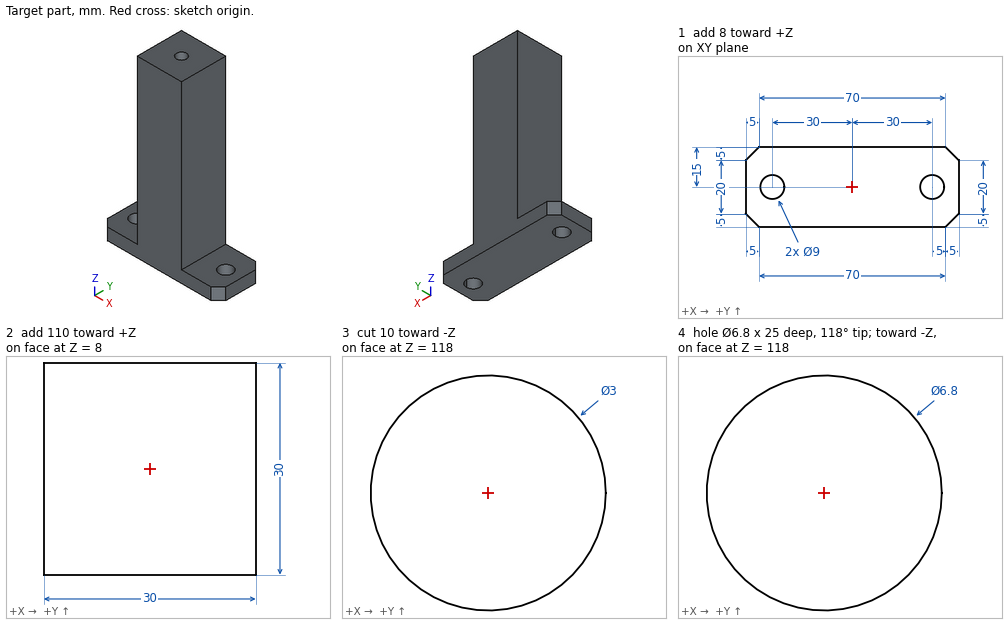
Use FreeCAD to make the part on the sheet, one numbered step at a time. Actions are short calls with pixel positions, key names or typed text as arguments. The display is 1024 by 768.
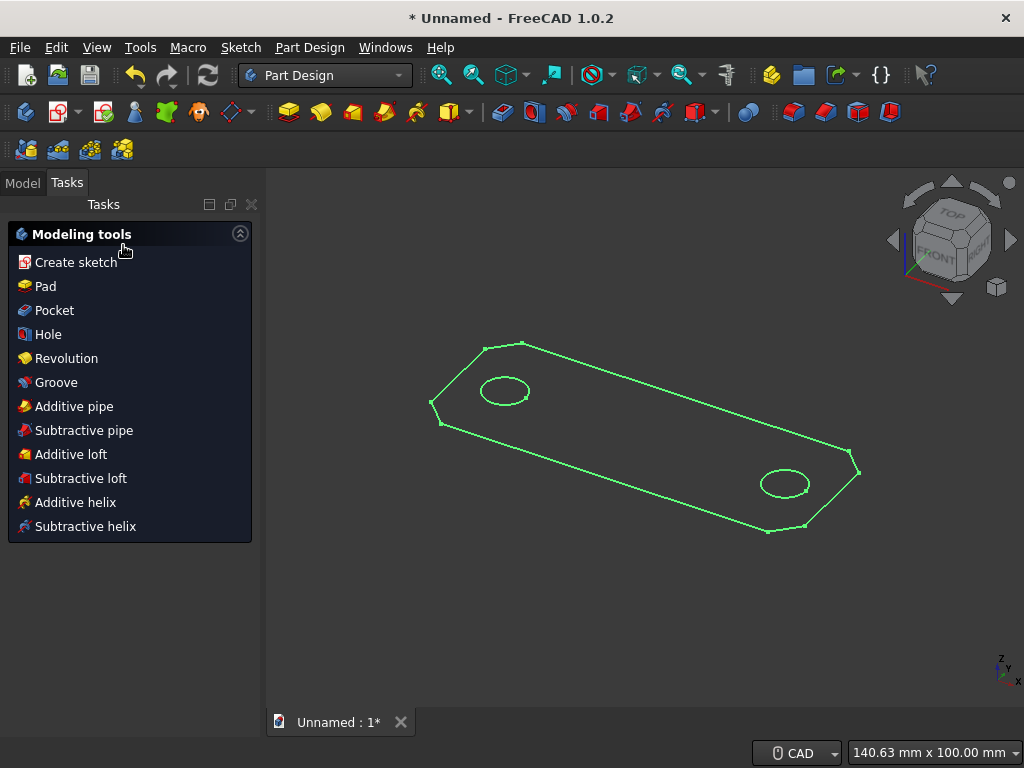
click(290, 112)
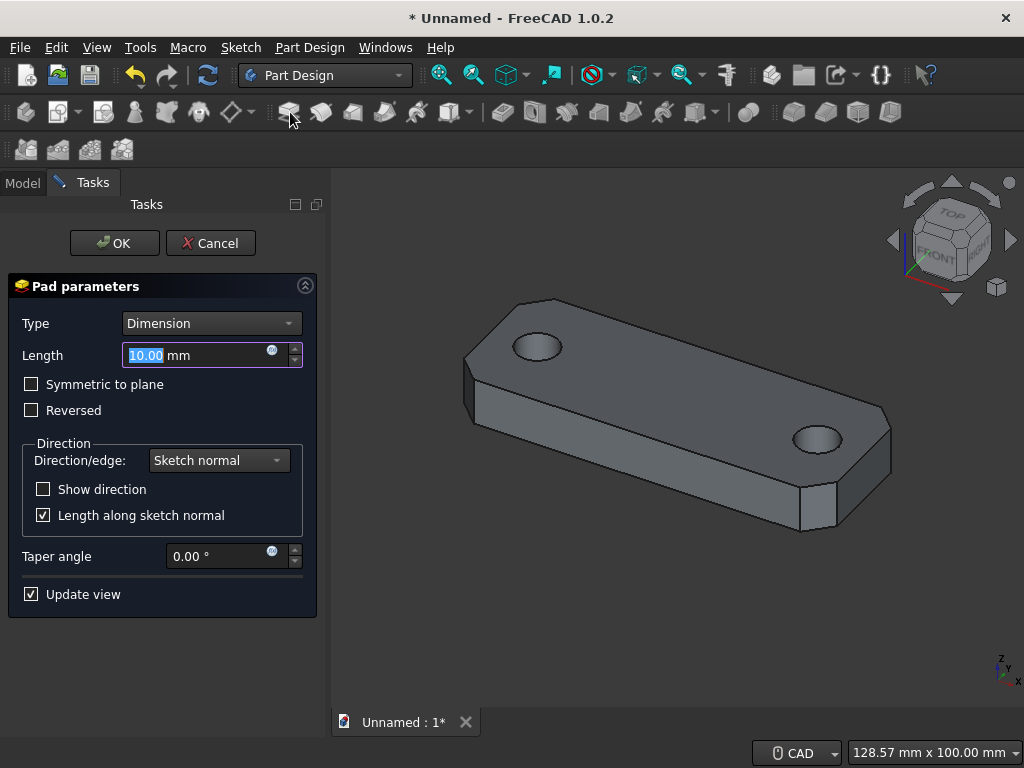
text(8)
key(Tab)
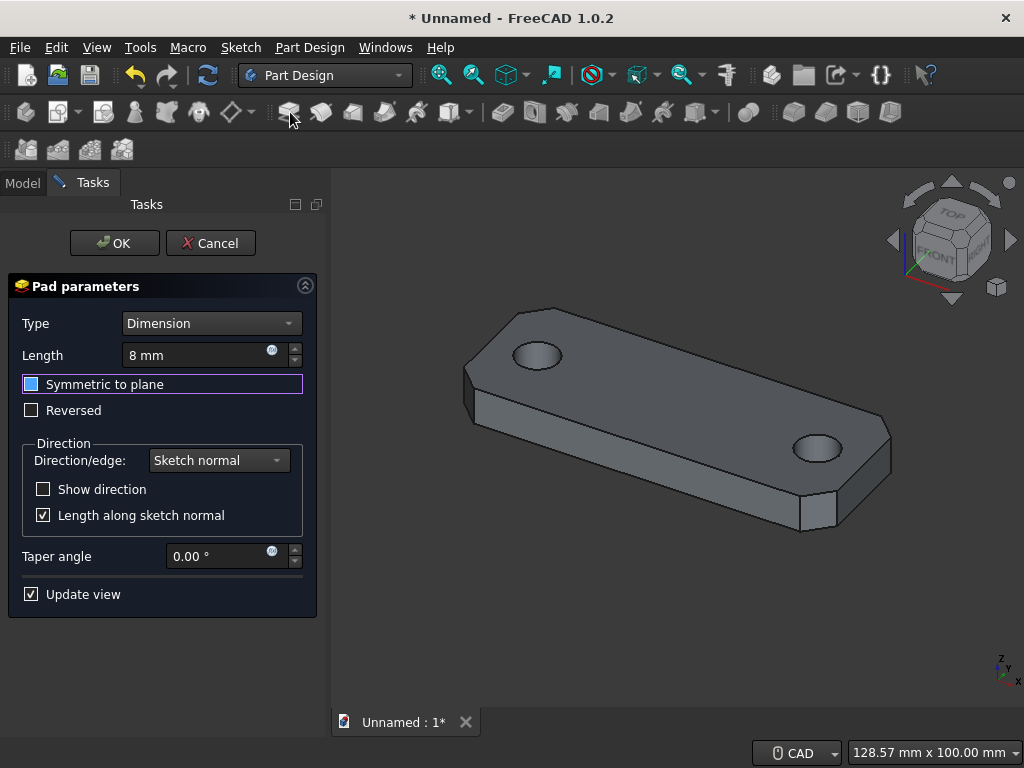
click(115, 243)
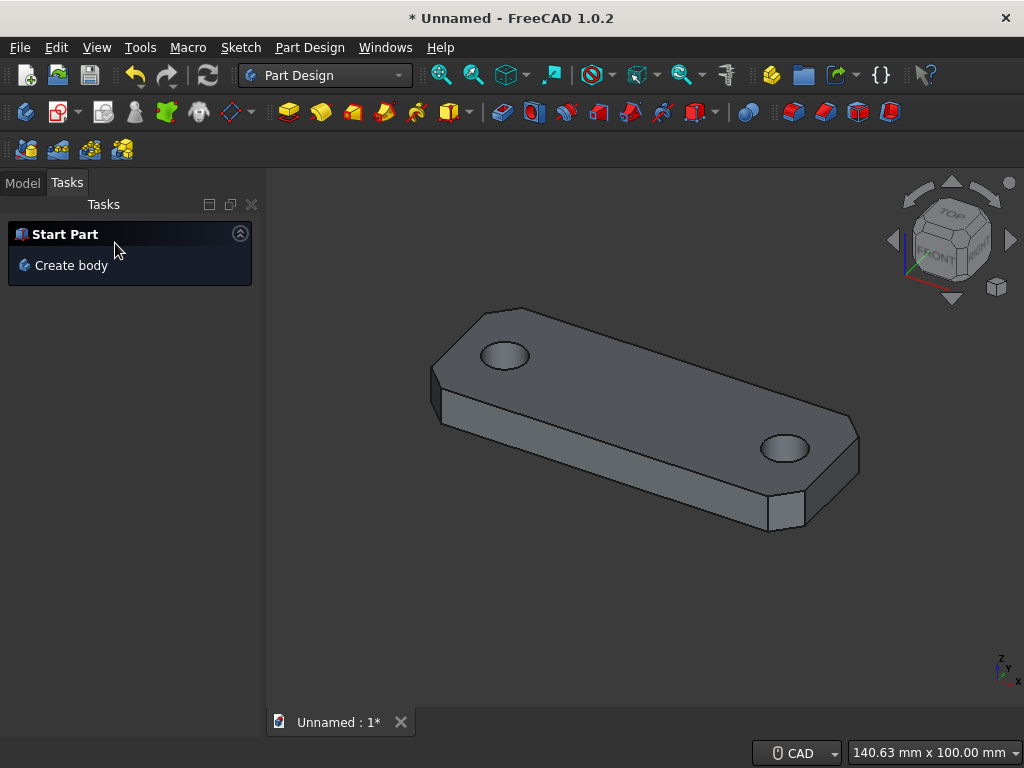
click(645, 401)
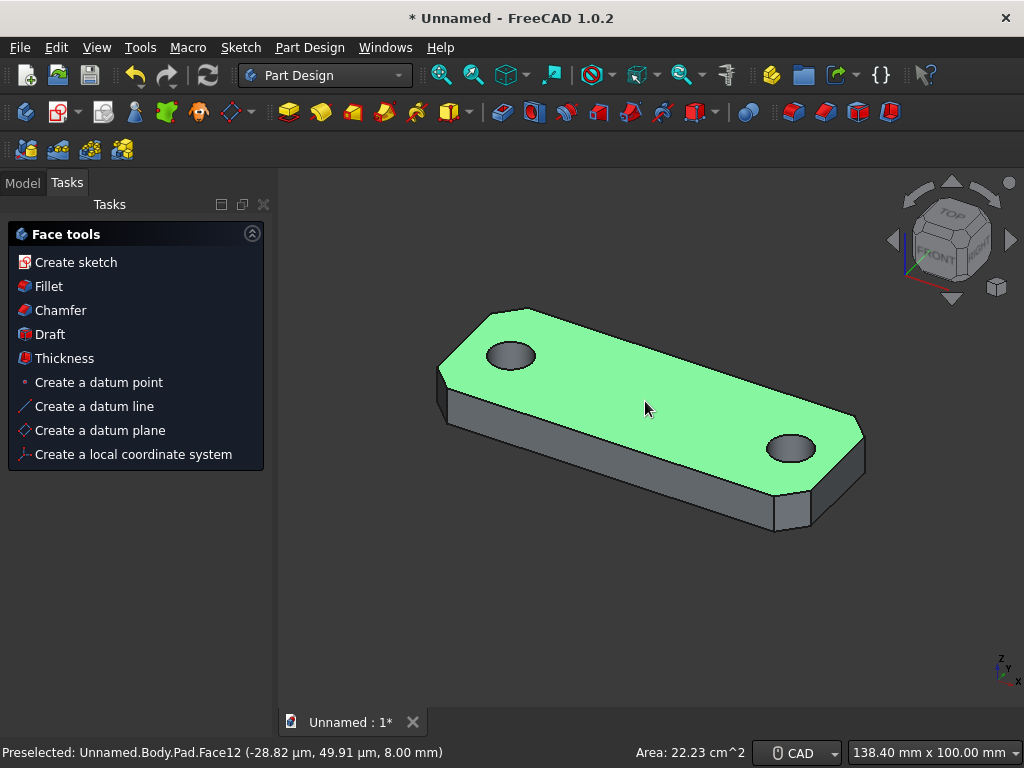
click(58, 112)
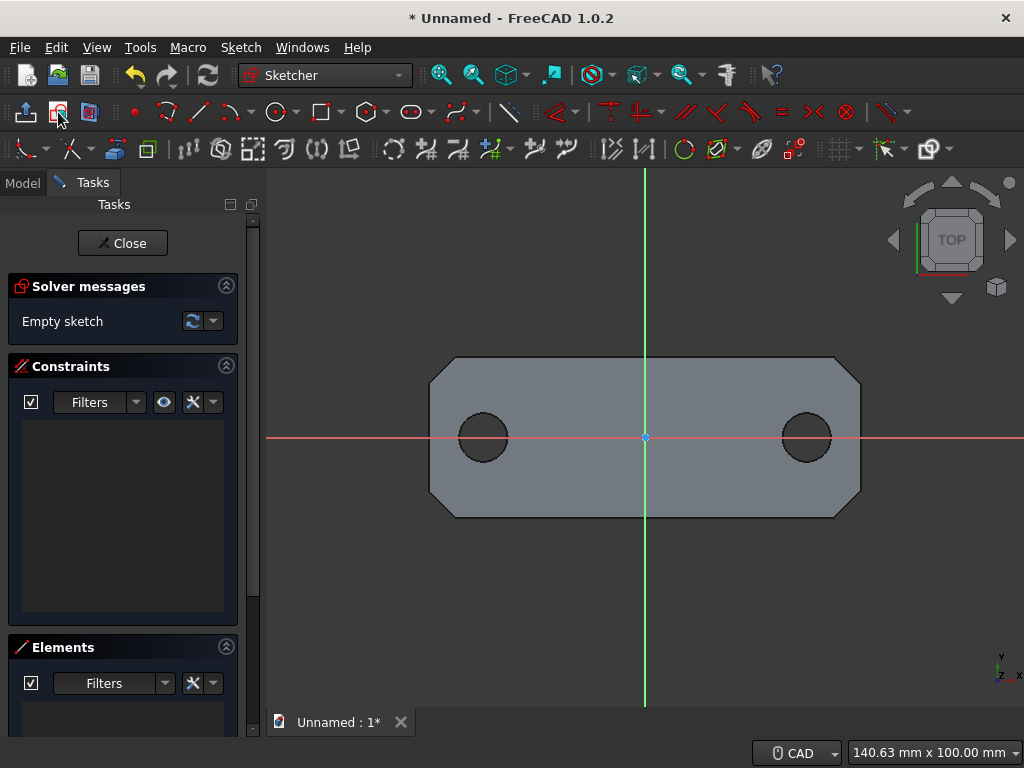
scroll(701, 438, up, 4)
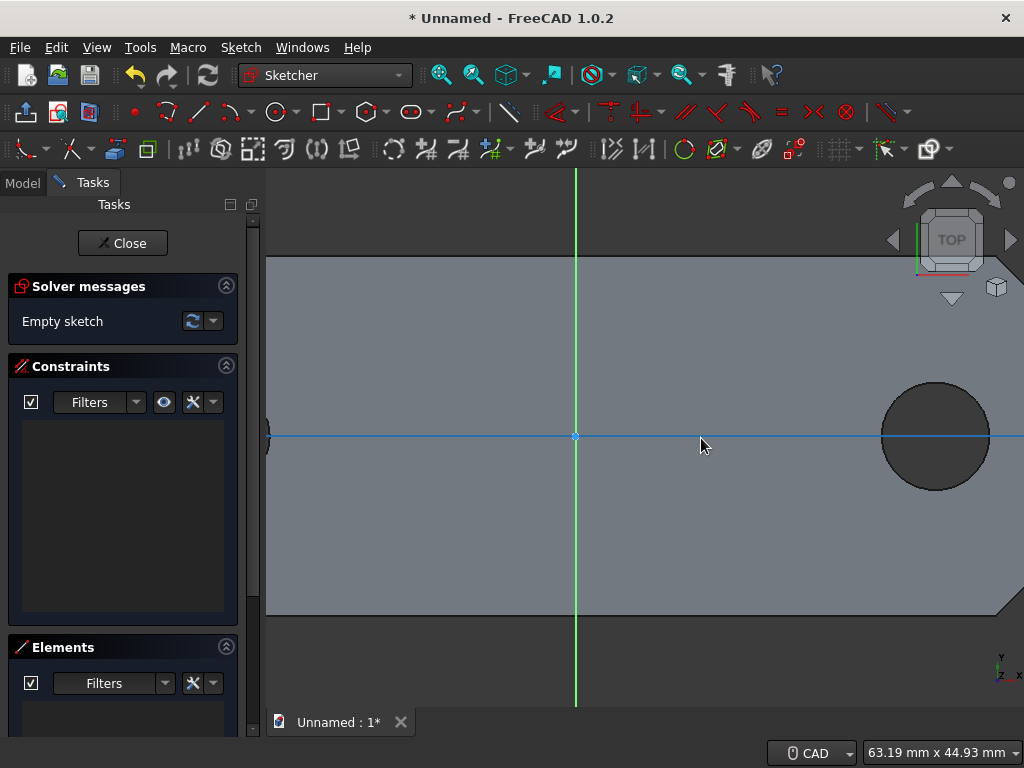
click(344, 112)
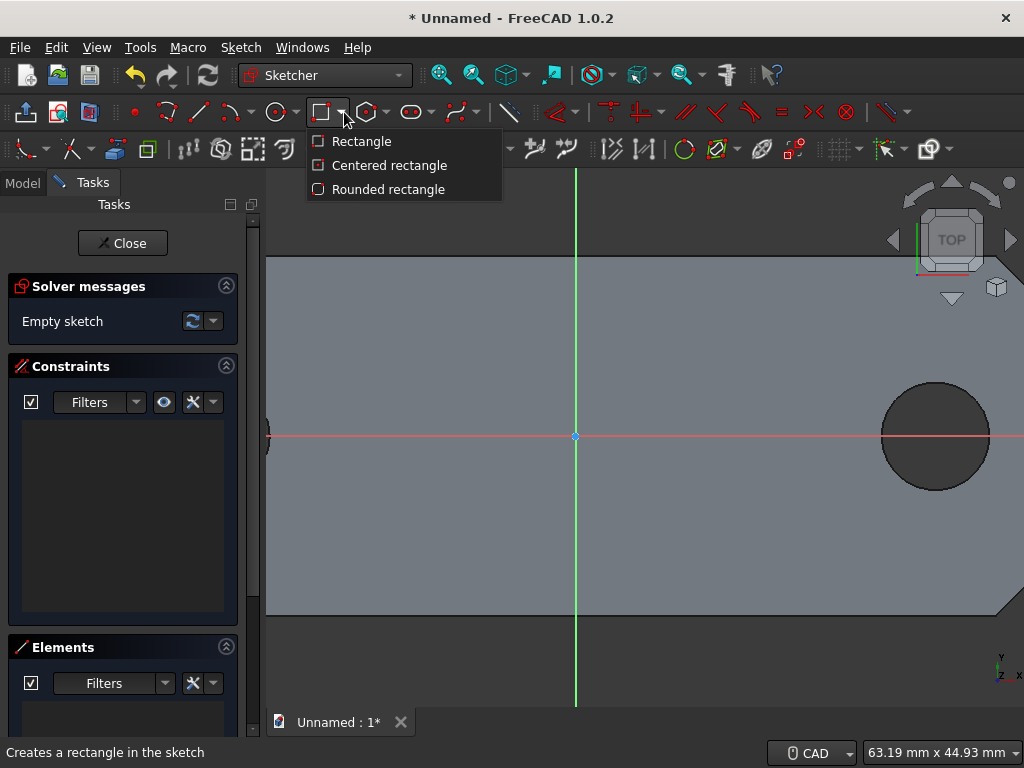
click(404, 165)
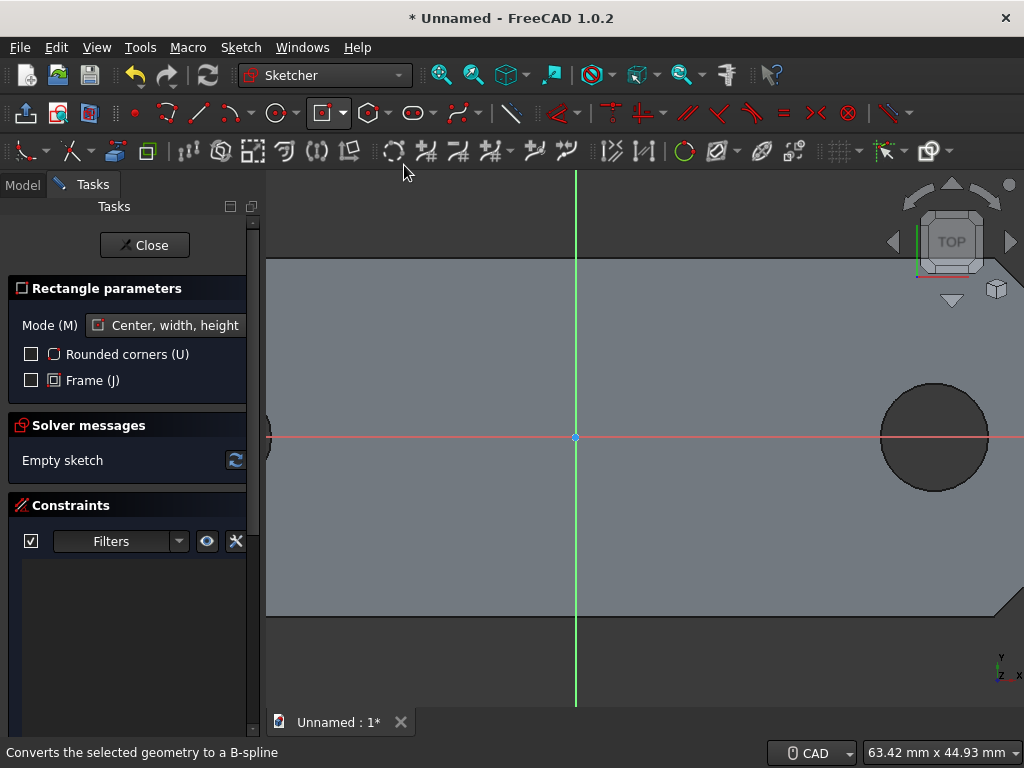
click(576, 437)
click(755, 258)
key(Escape)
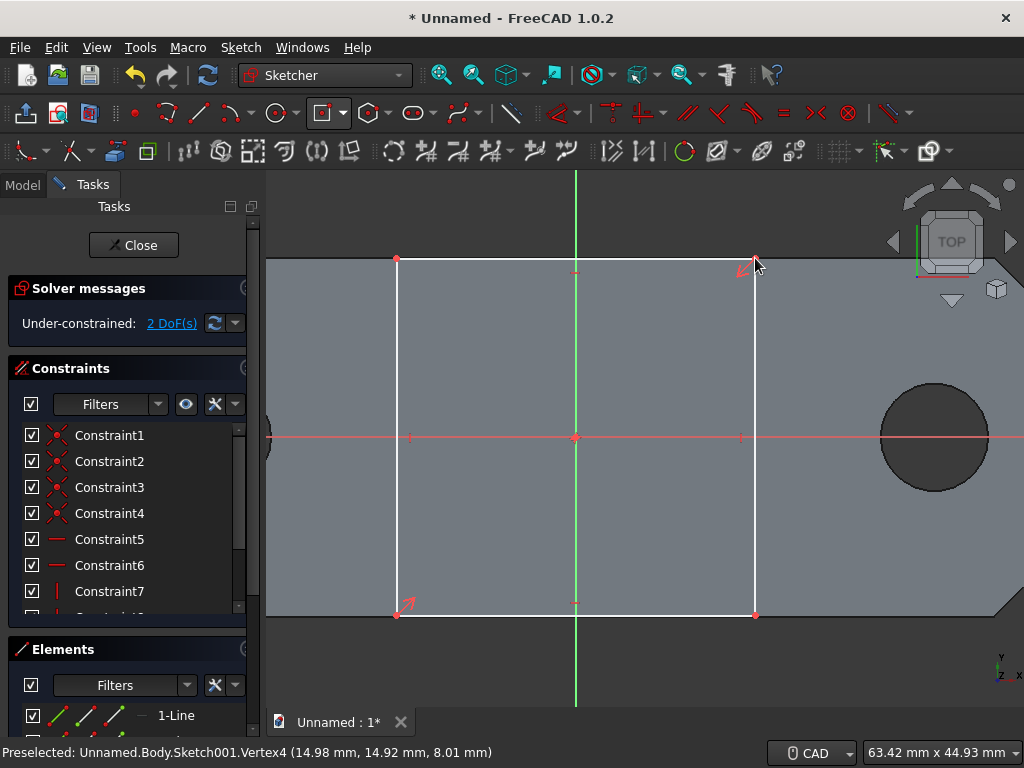
click(558, 114)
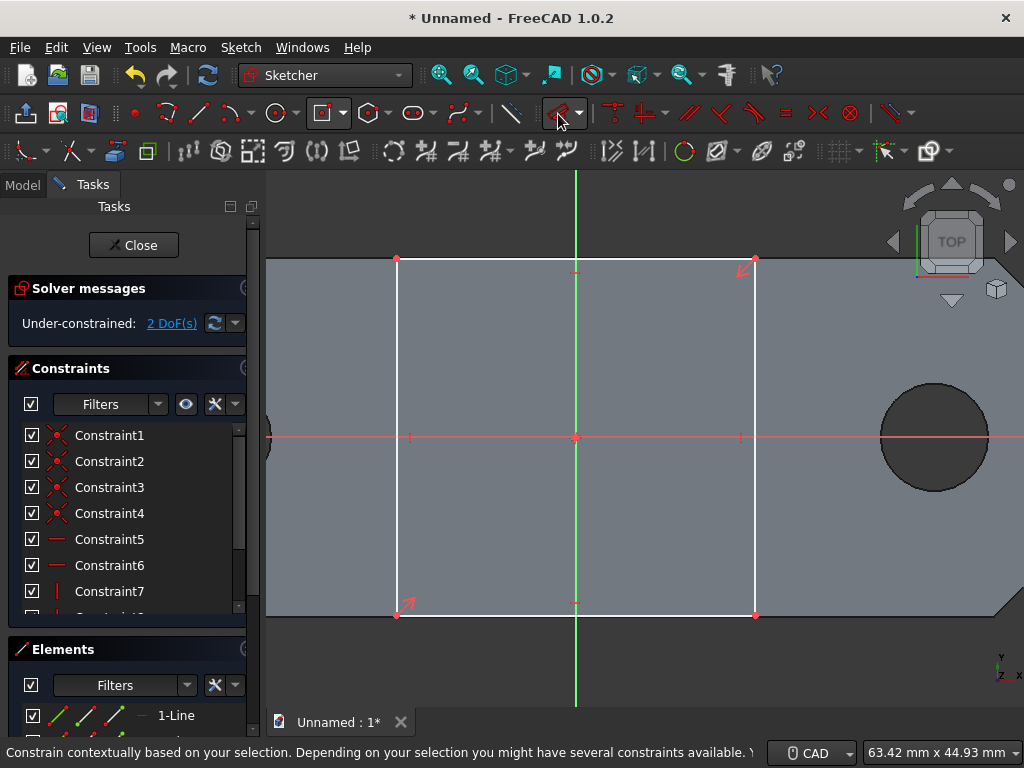
click(504, 616)
click(494, 650)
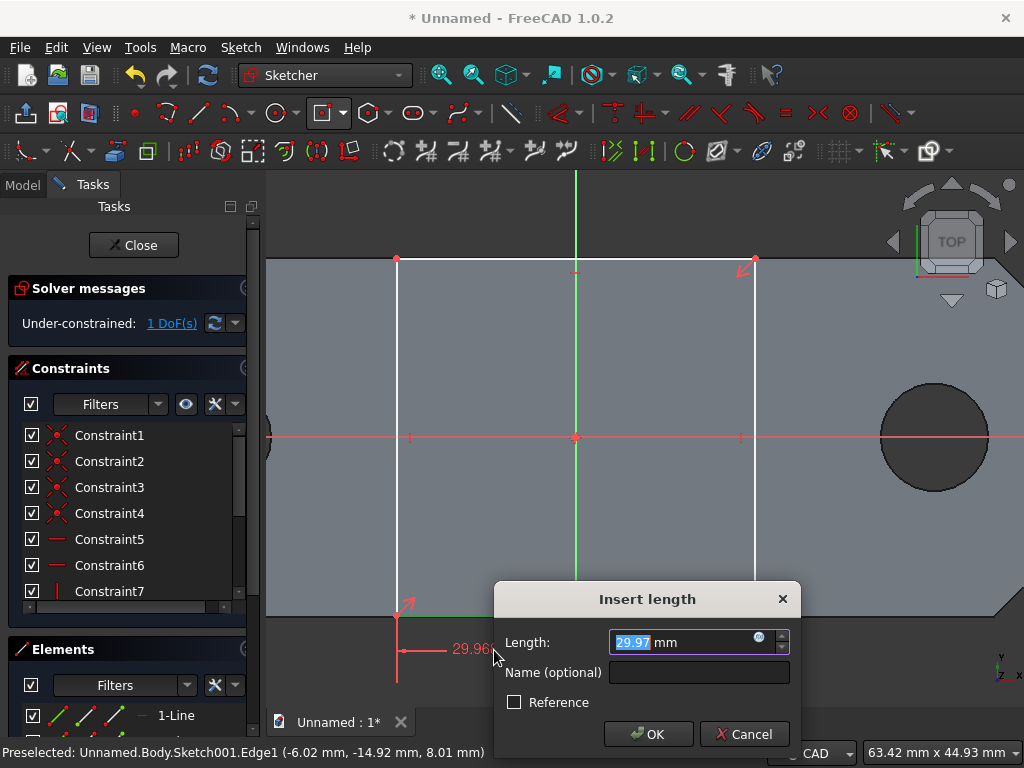
text(30)
key(Return)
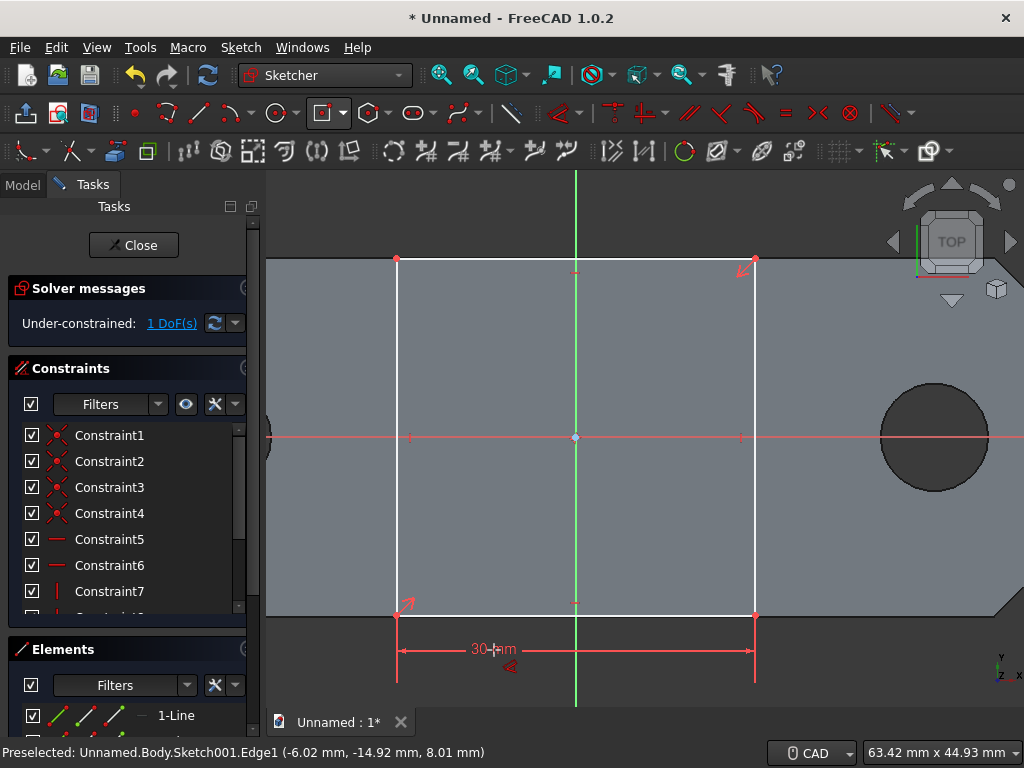
click(755, 509)
click(789, 355)